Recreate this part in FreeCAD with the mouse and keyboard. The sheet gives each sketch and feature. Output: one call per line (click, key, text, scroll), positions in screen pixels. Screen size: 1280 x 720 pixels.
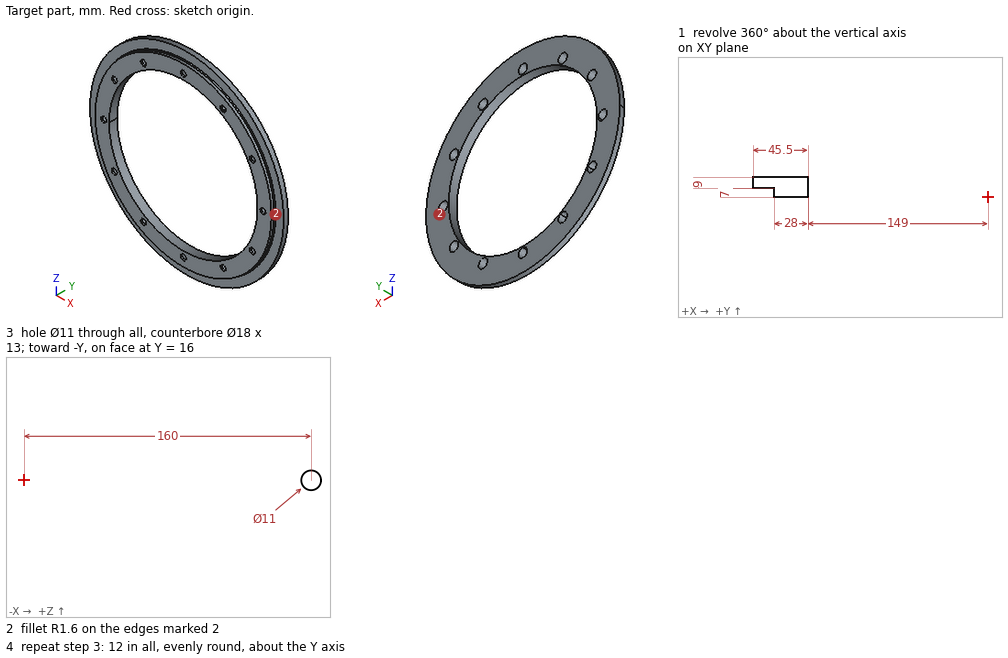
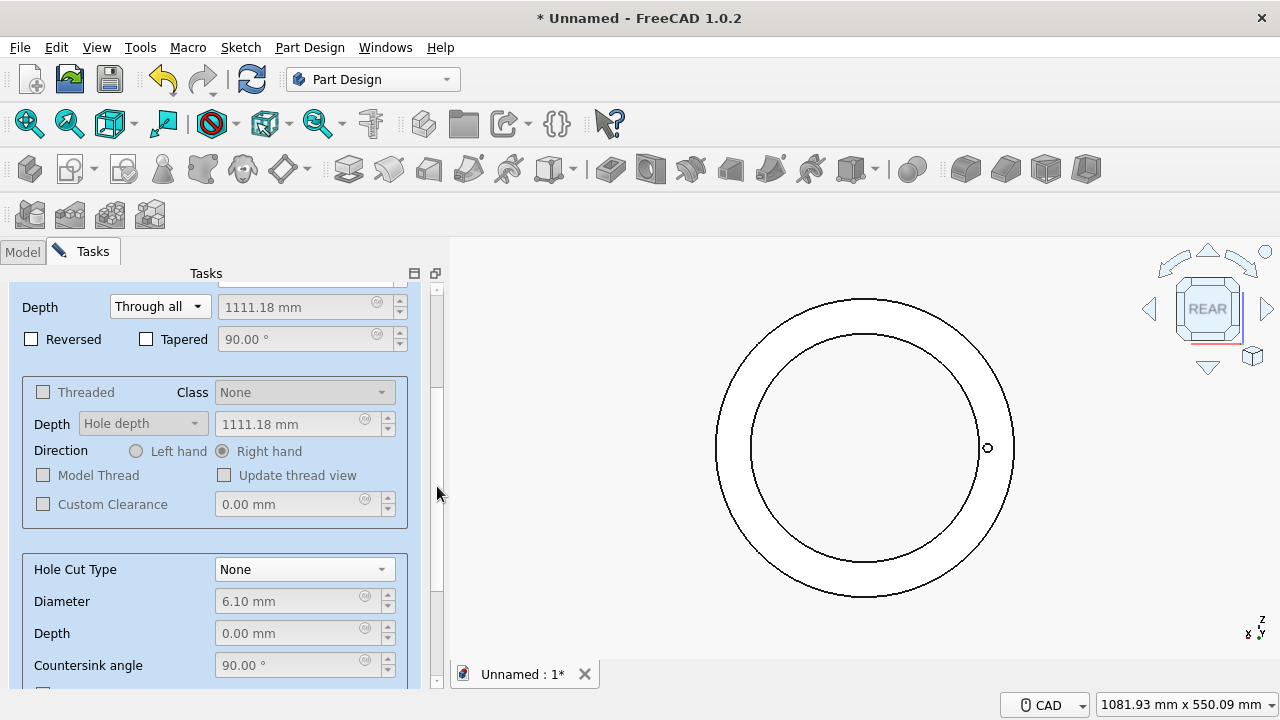
click(306, 570)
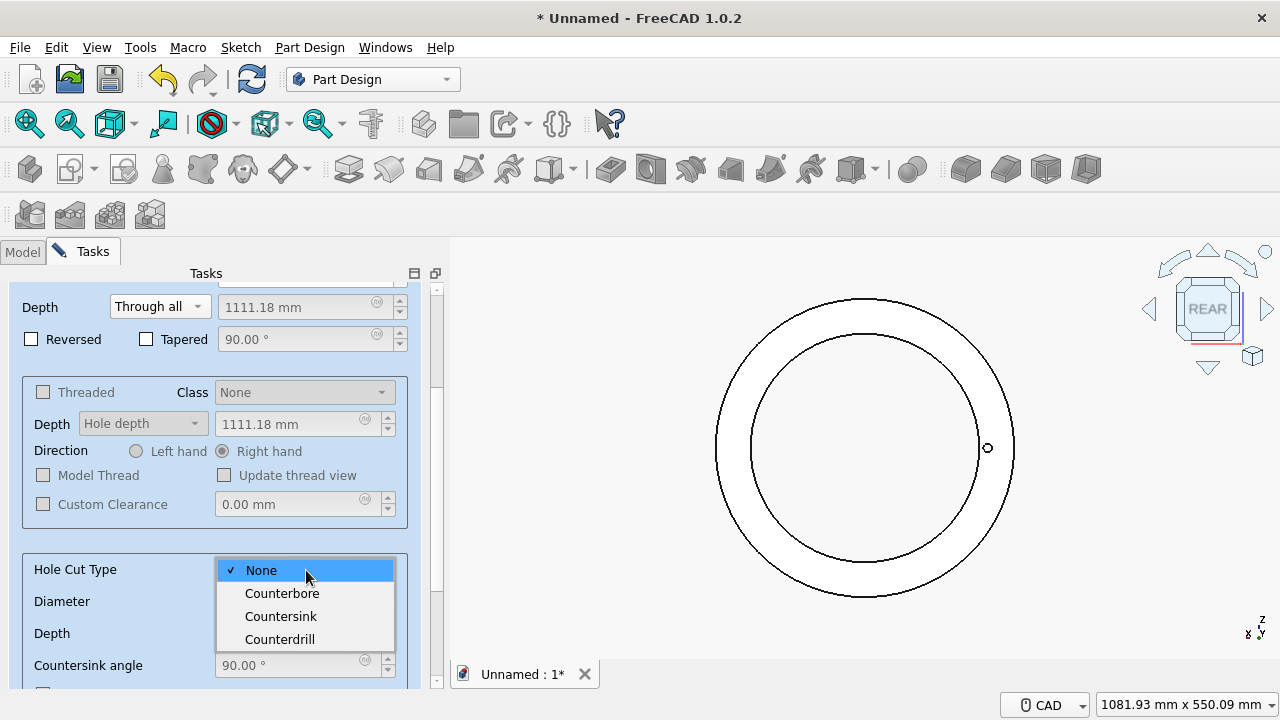
click(304, 594)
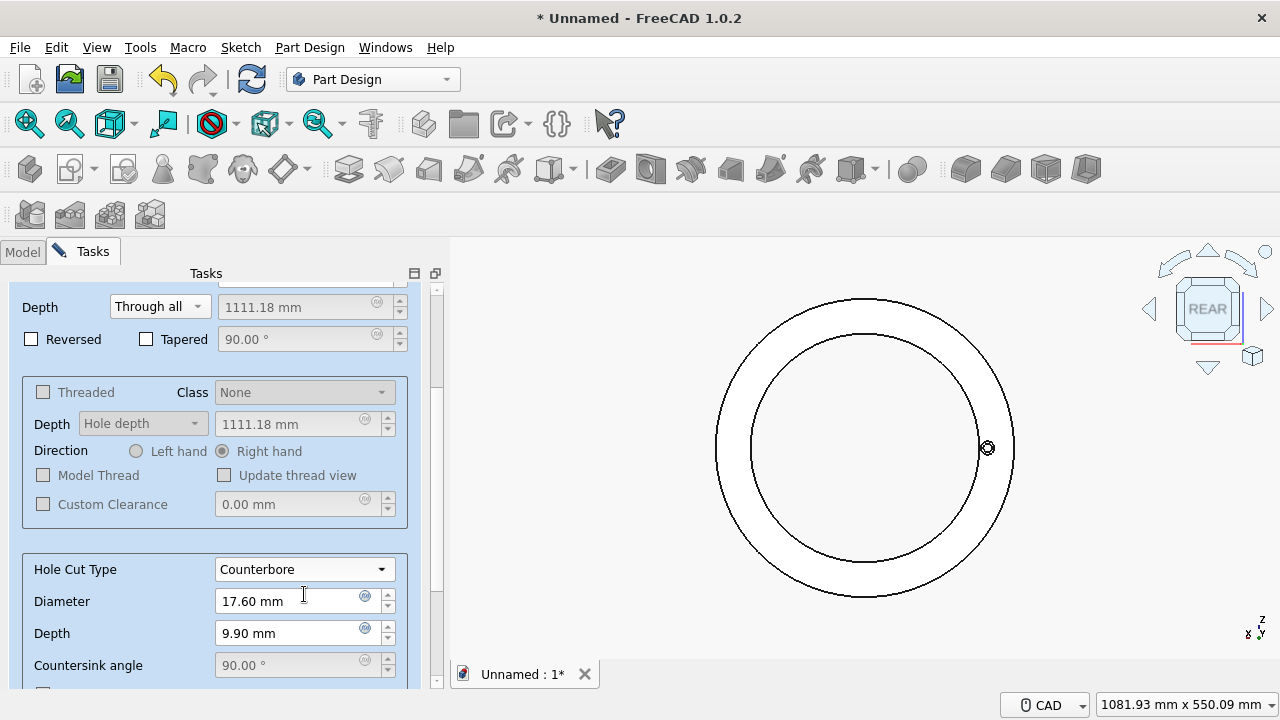
triple_click(298, 601)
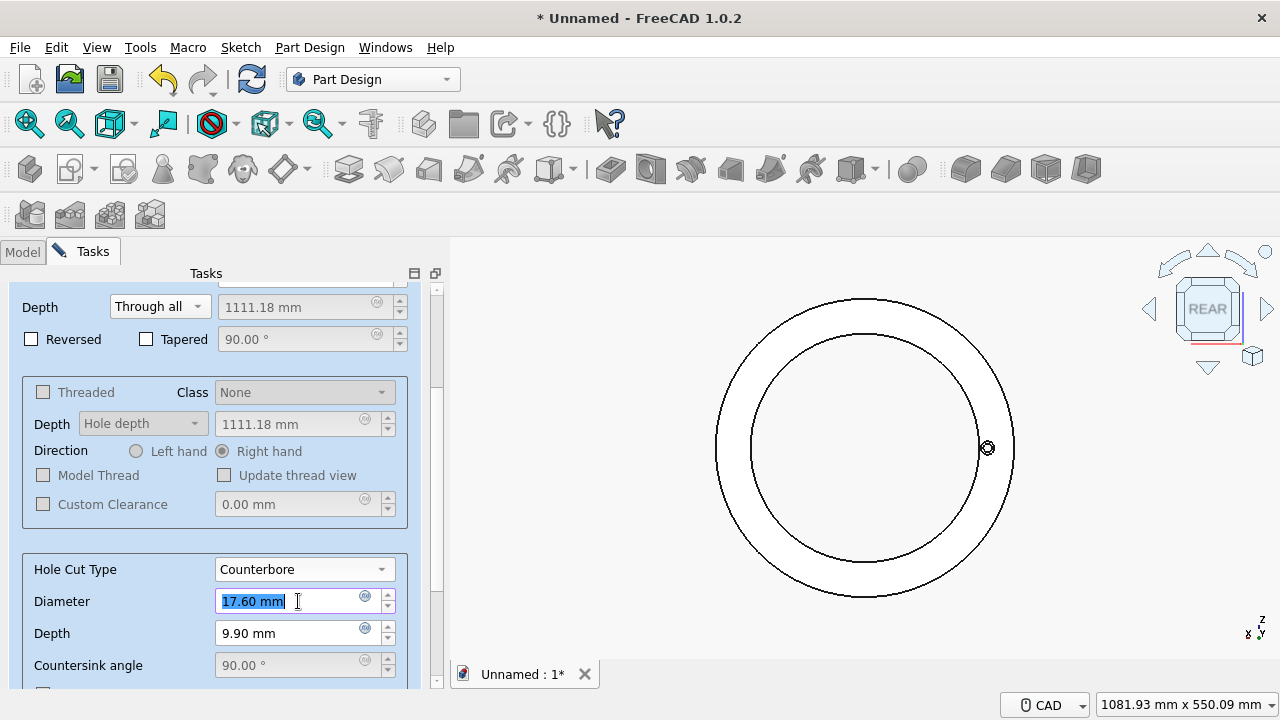
text(18)
key(Tab)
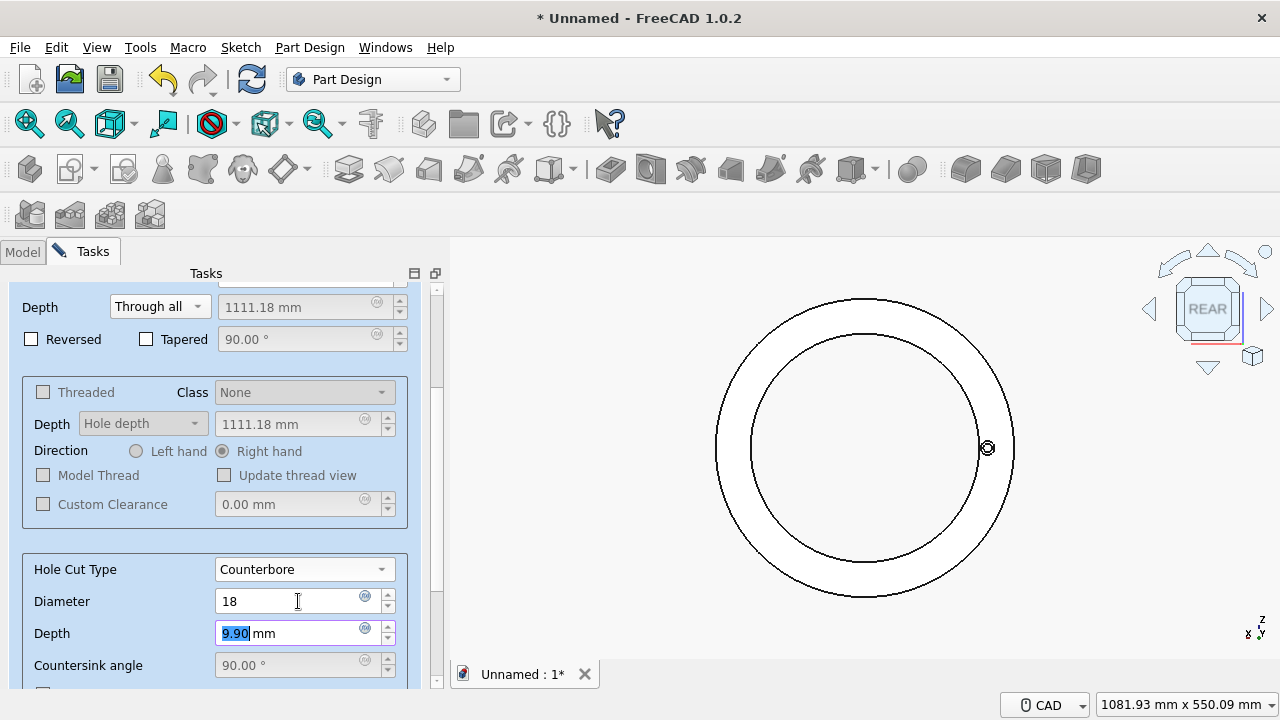
text(13)
key(Tab)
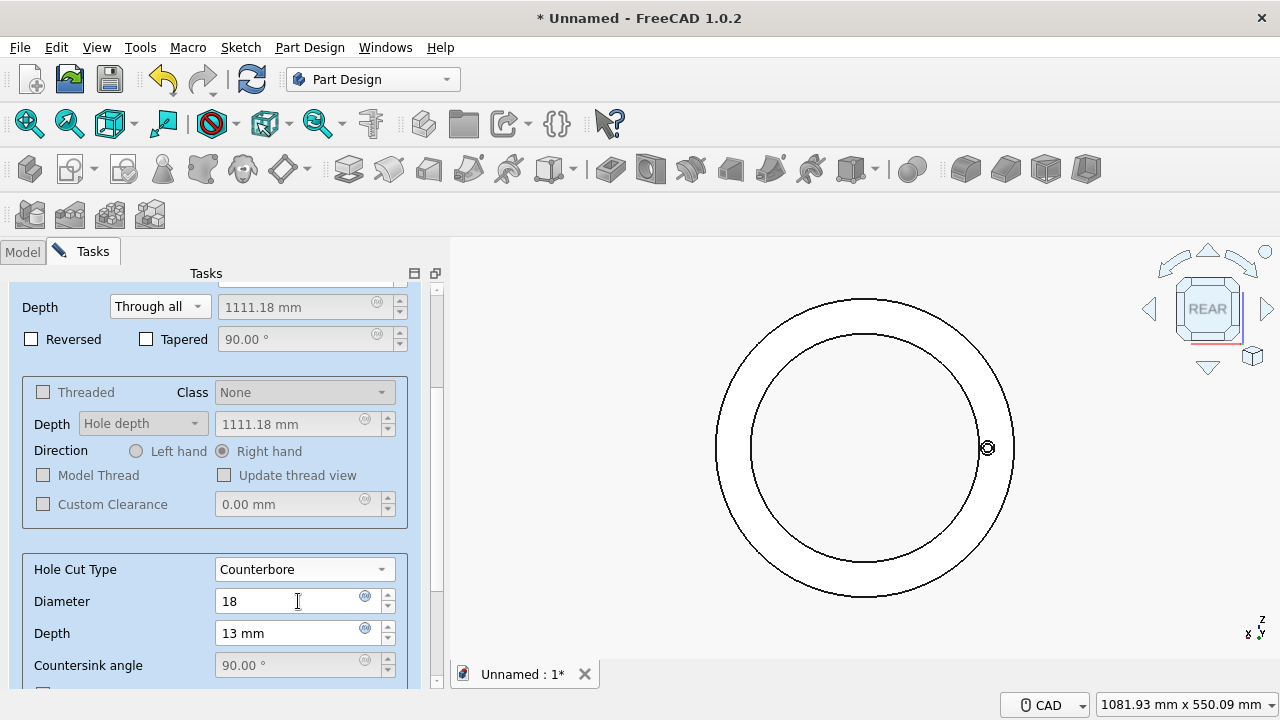
scroll(437, 486, up, 4)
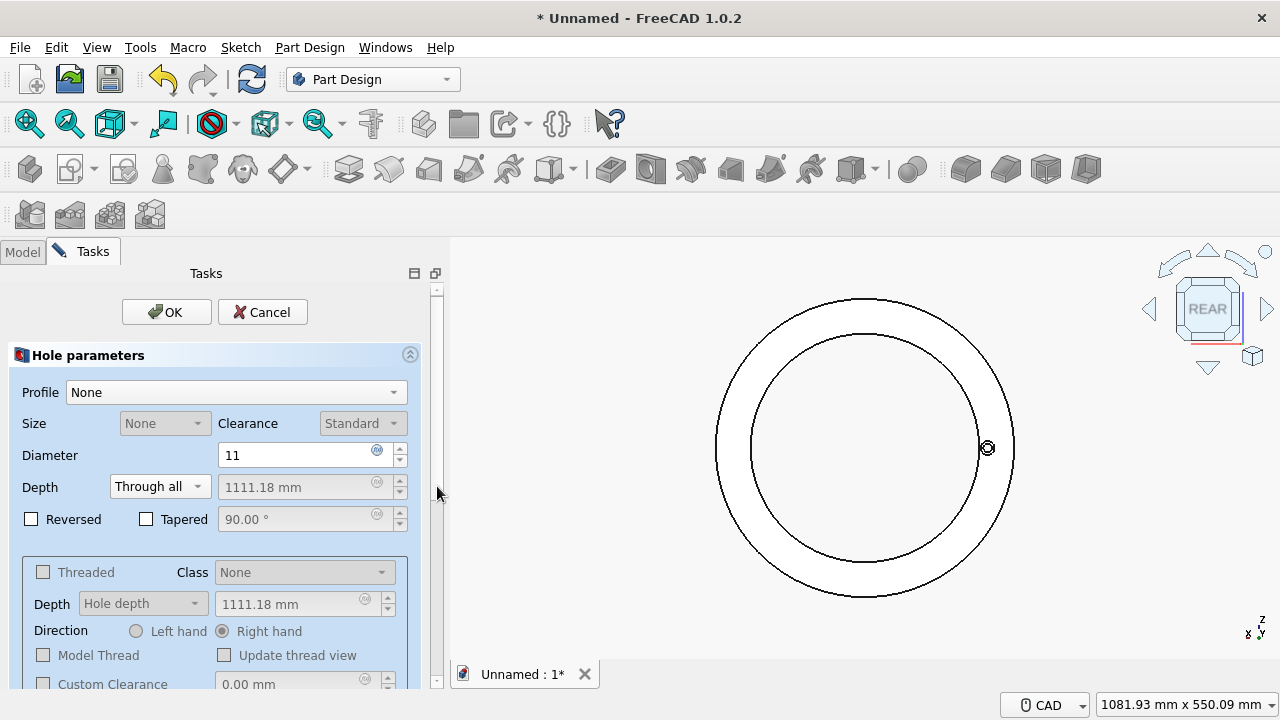
click(167, 312)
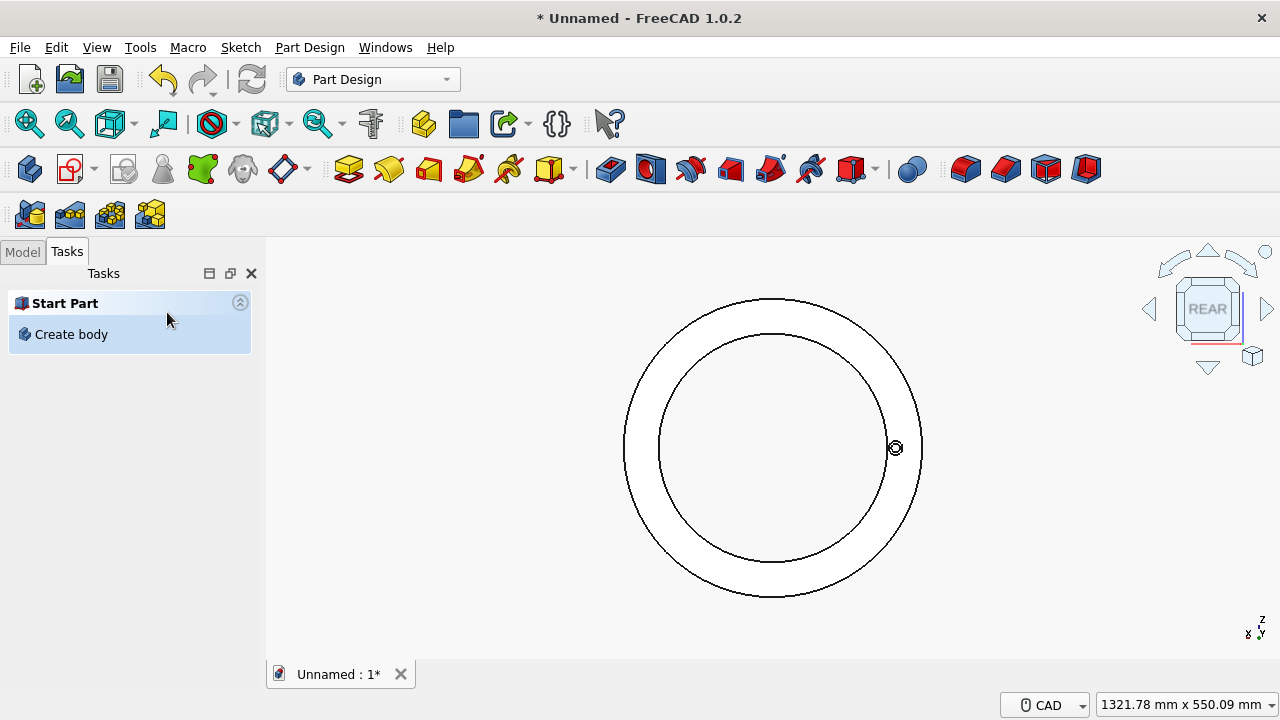
click(23, 251)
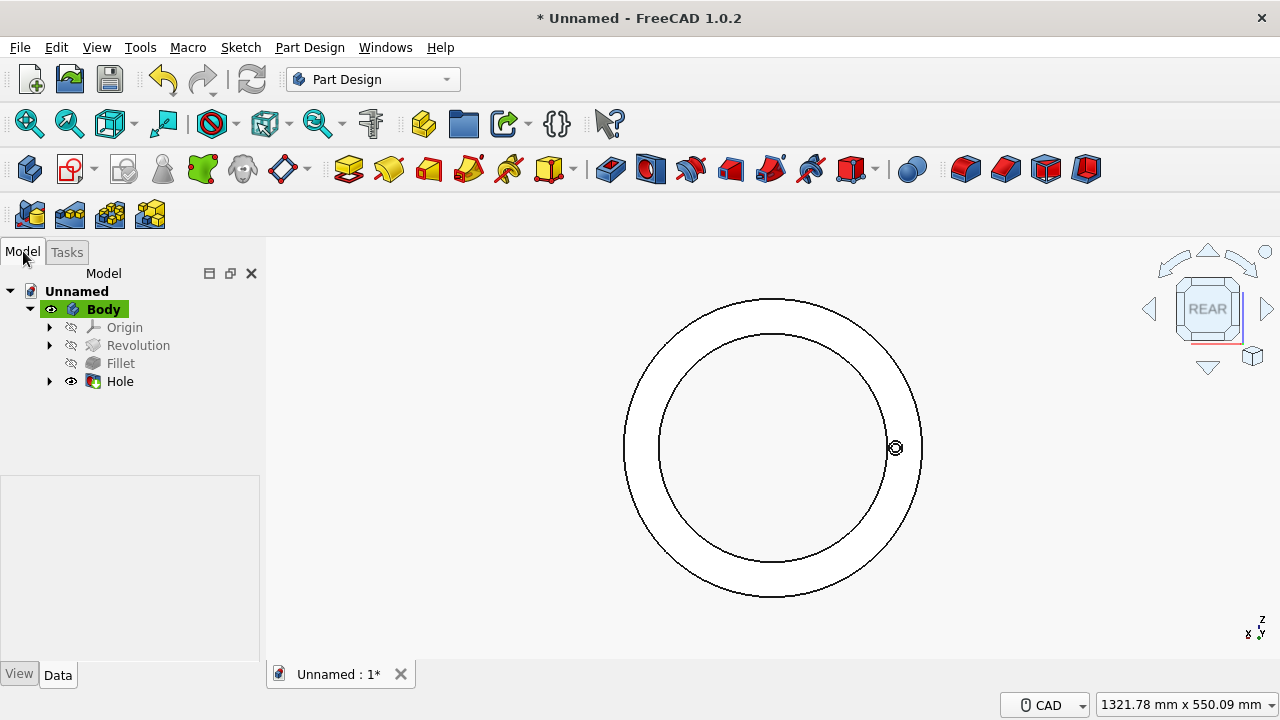
click(116, 381)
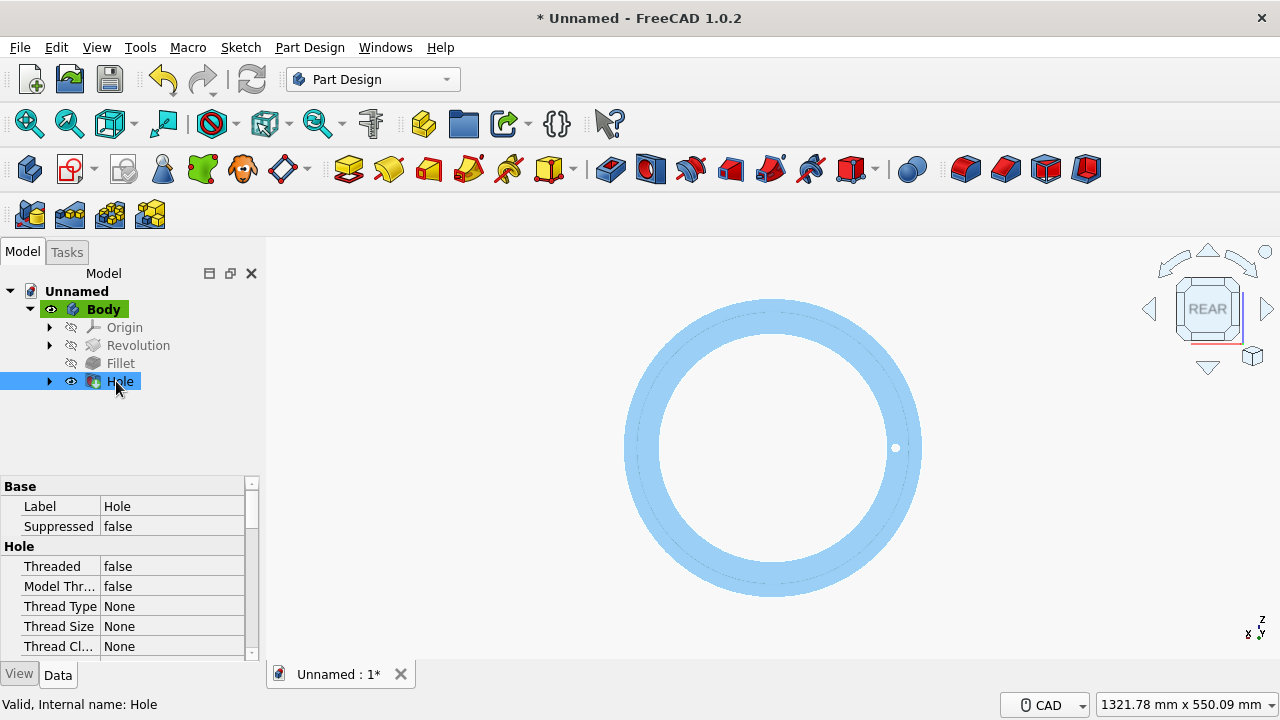
click(110, 214)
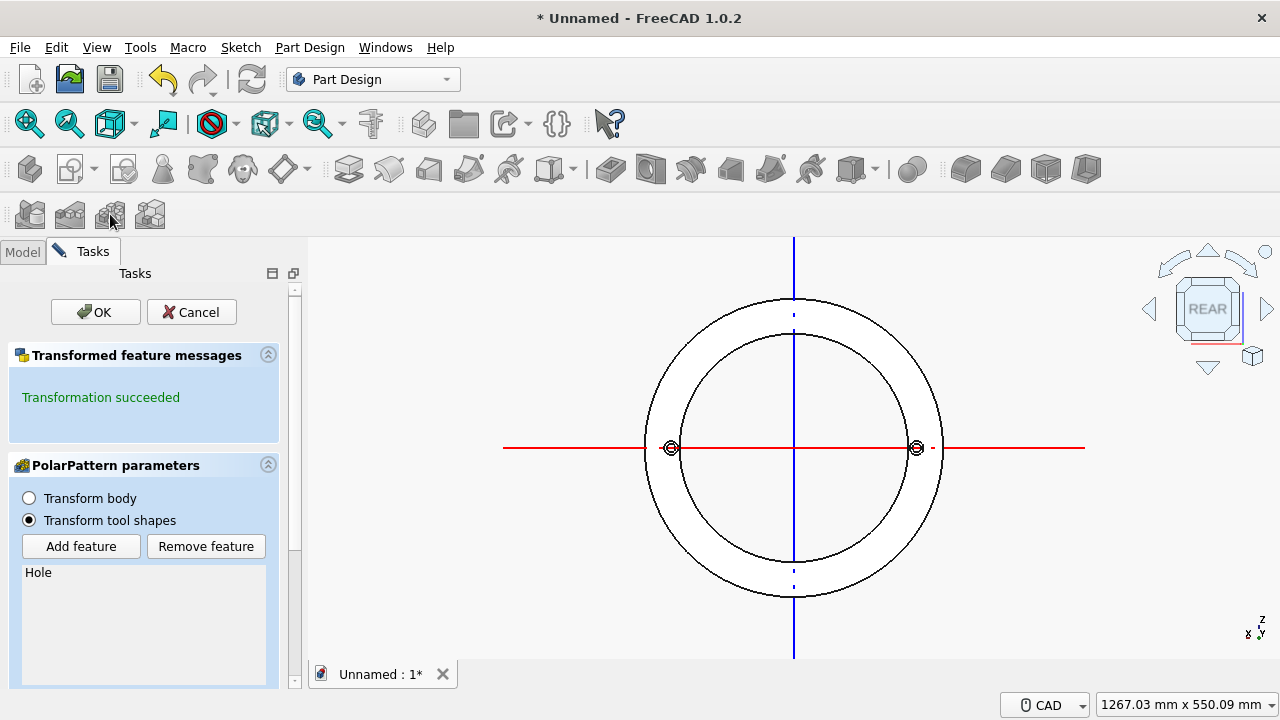
scroll(295, 486, down, 2)